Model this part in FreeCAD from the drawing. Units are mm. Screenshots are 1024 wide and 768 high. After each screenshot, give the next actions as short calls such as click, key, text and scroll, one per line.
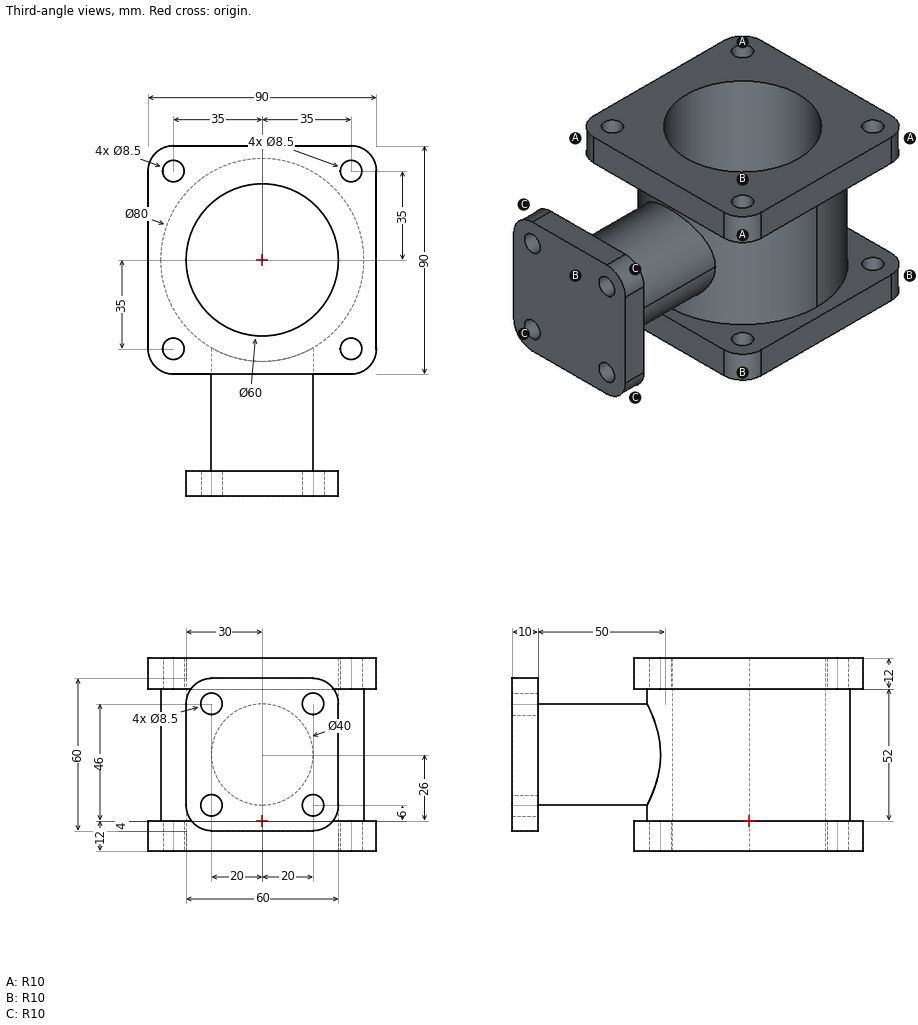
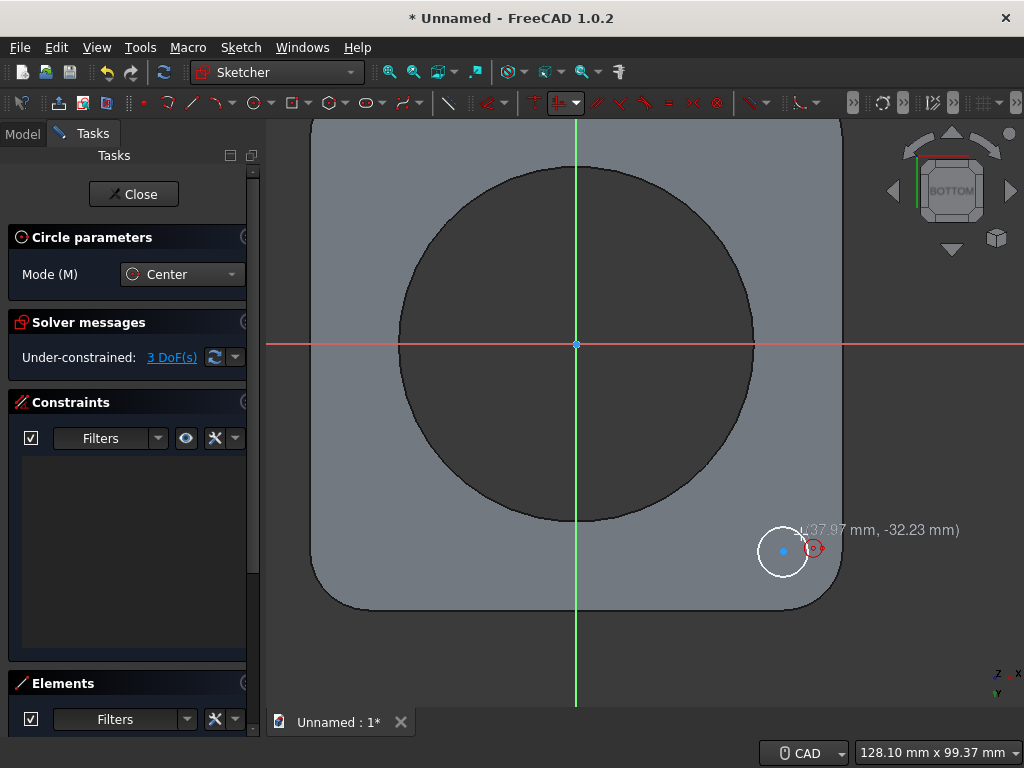
click(369, 551)
click(387, 534)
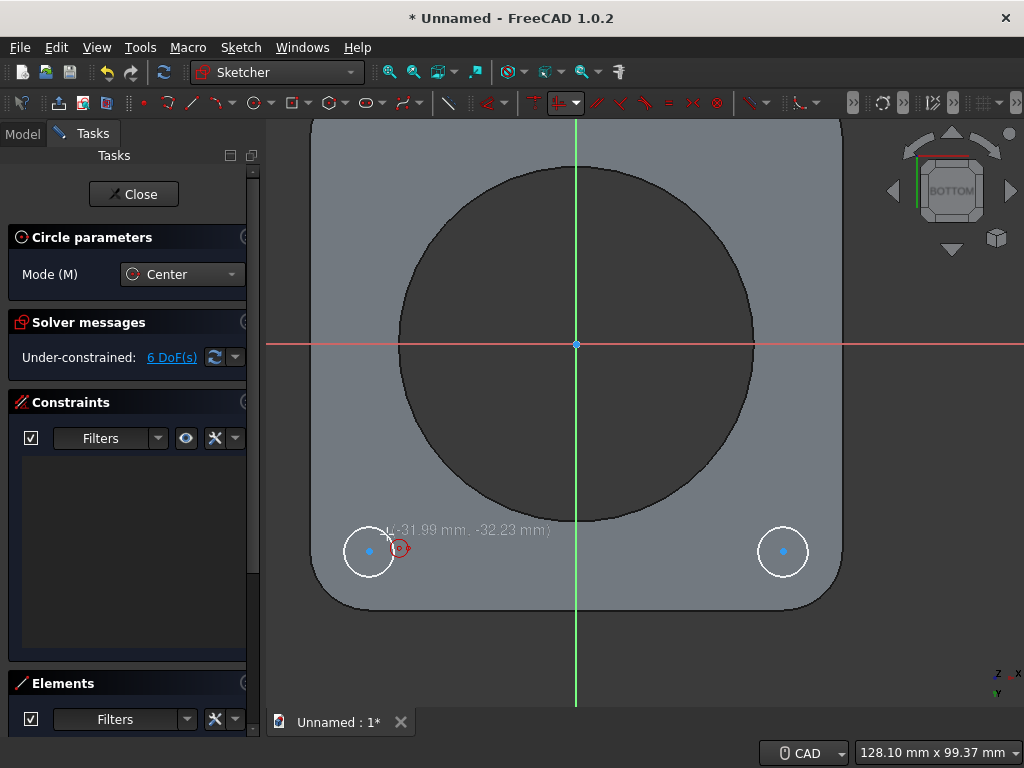
scroll(577, 679, down, 1)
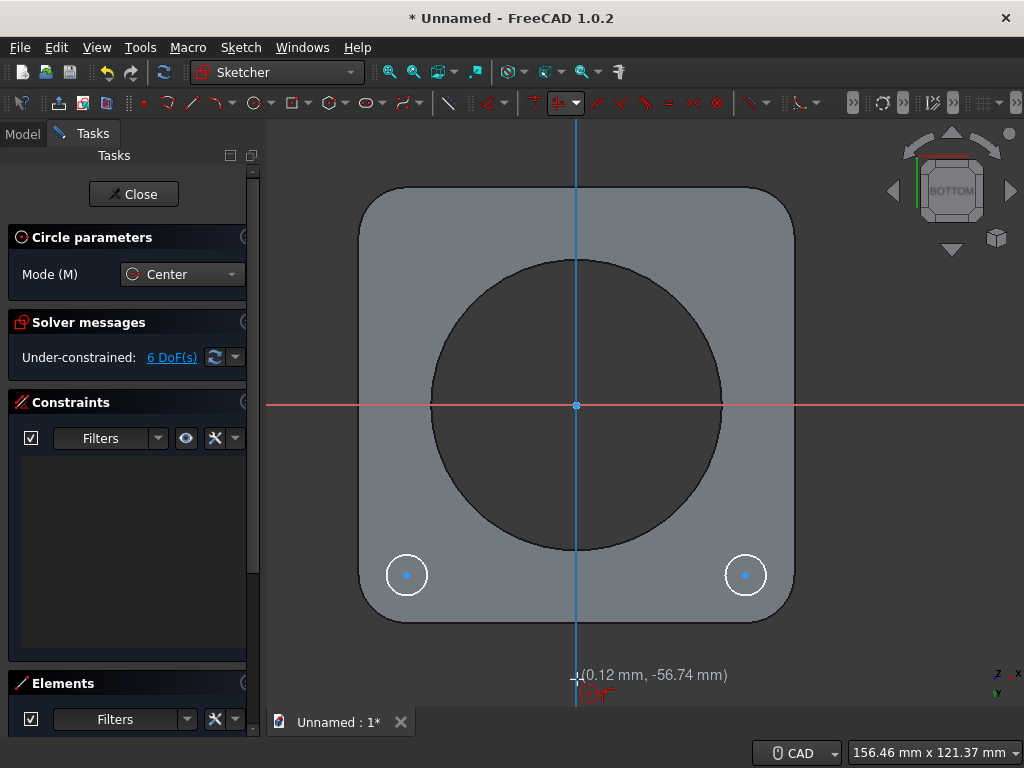
click(407, 236)
click(421, 221)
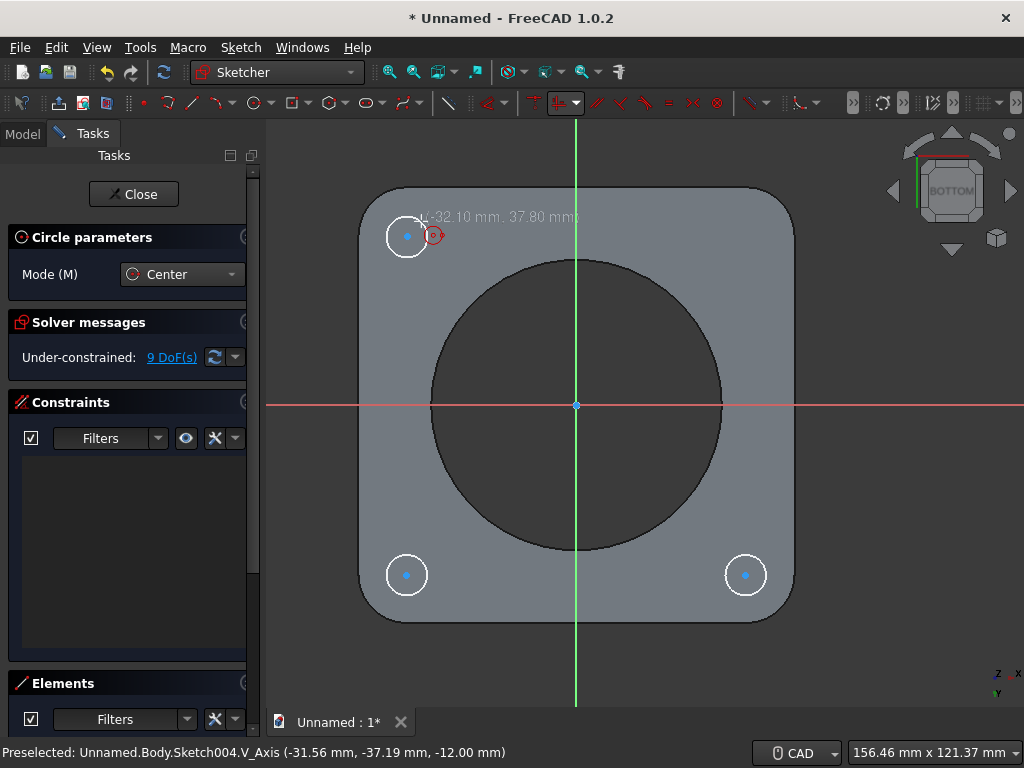
click(746, 236)
click(761, 221)
key(Escape)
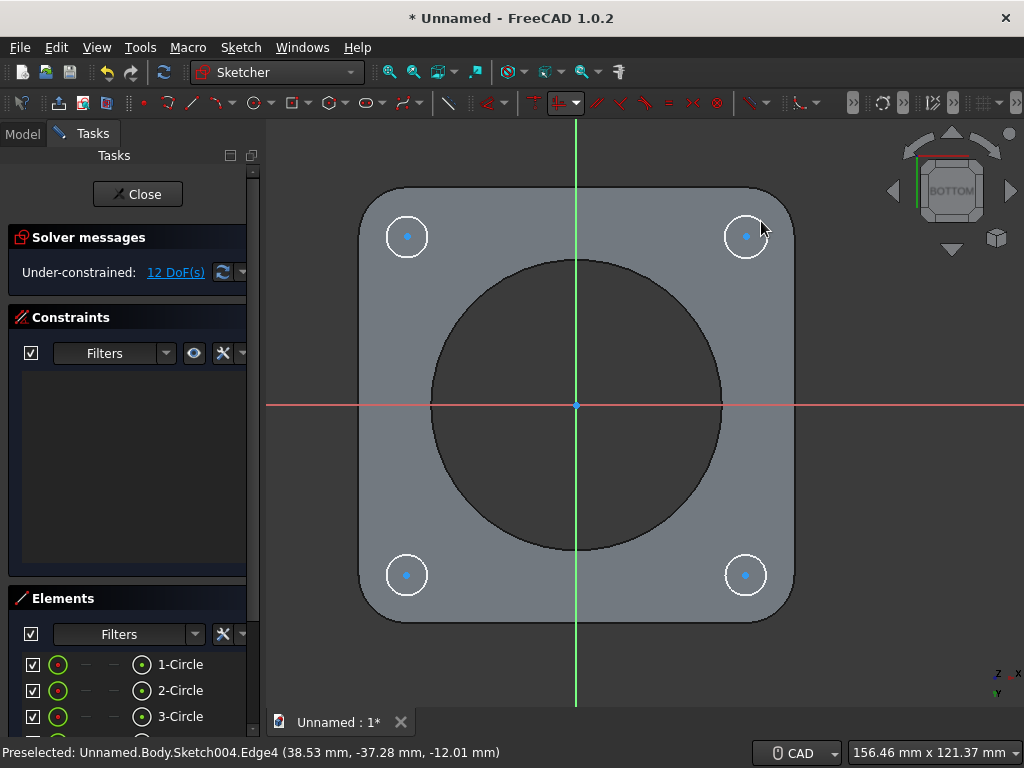
click(760, 561)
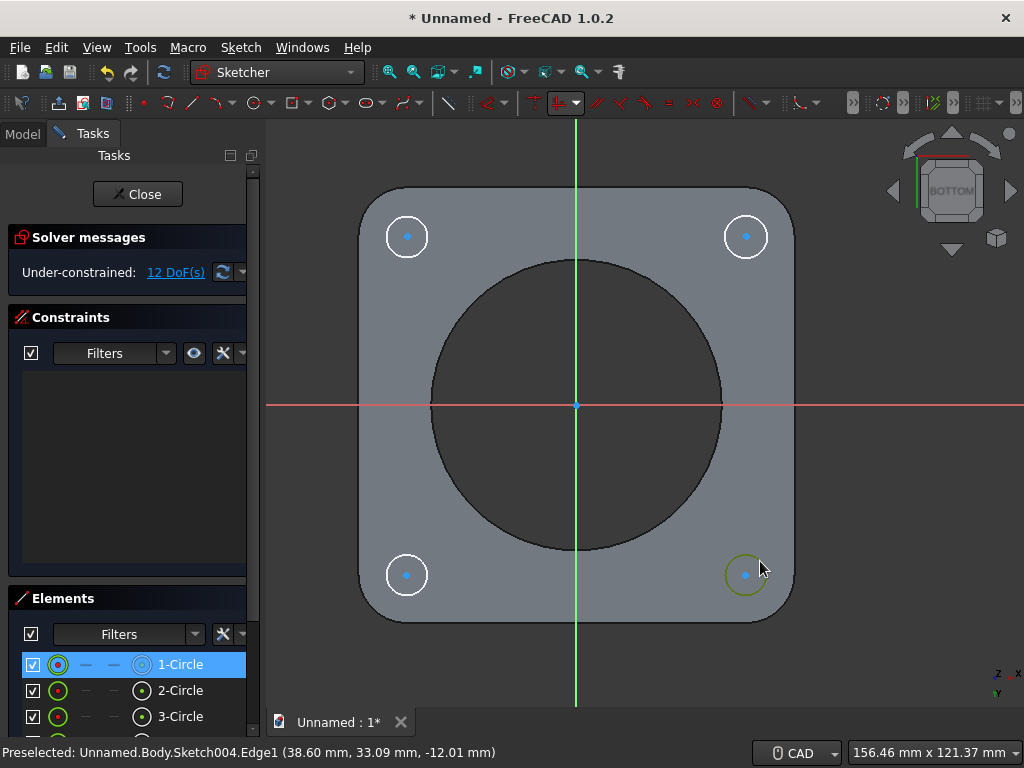
click(421, 561)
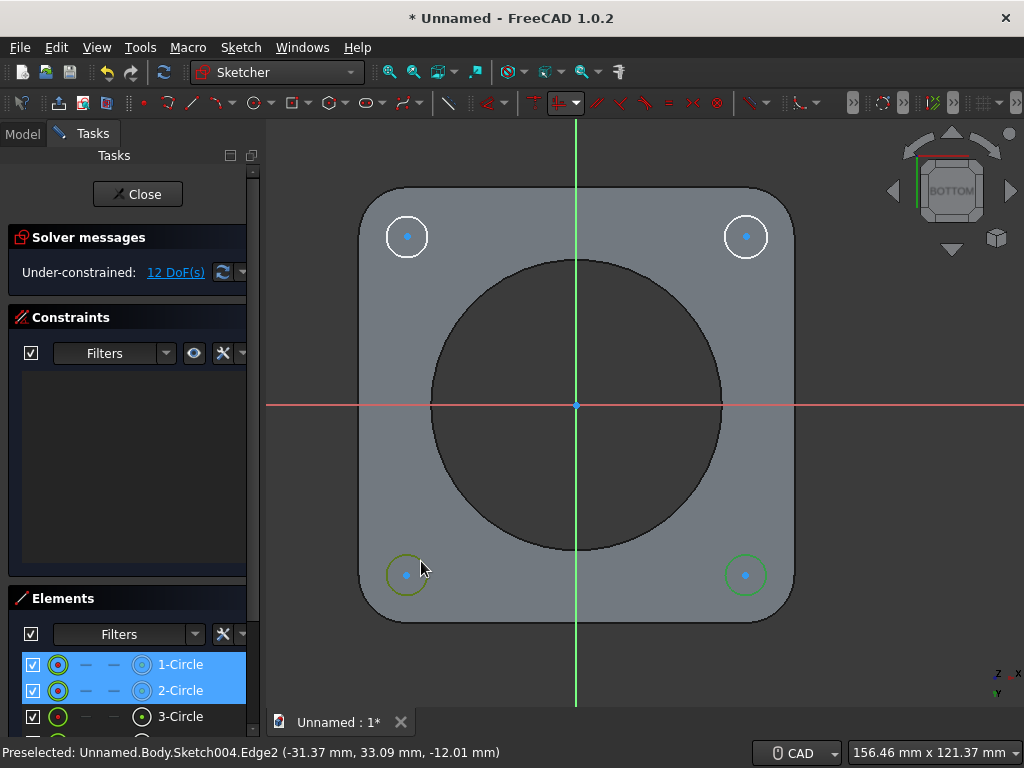
click(421, 222)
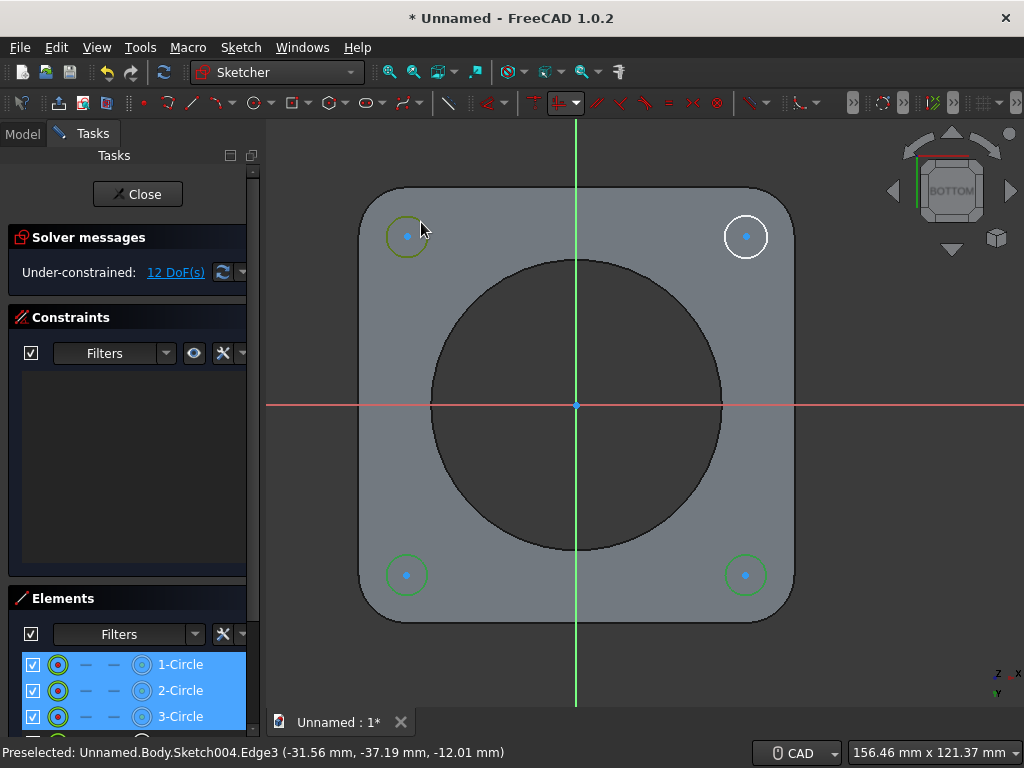
click(761, 222)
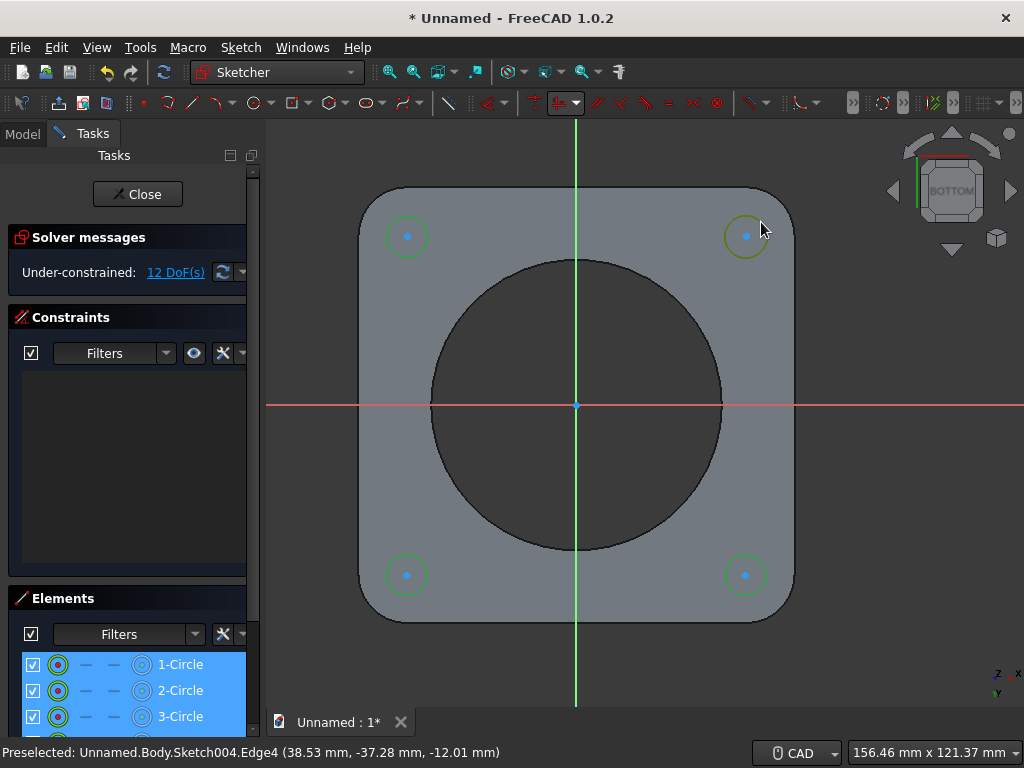
click(670, 104)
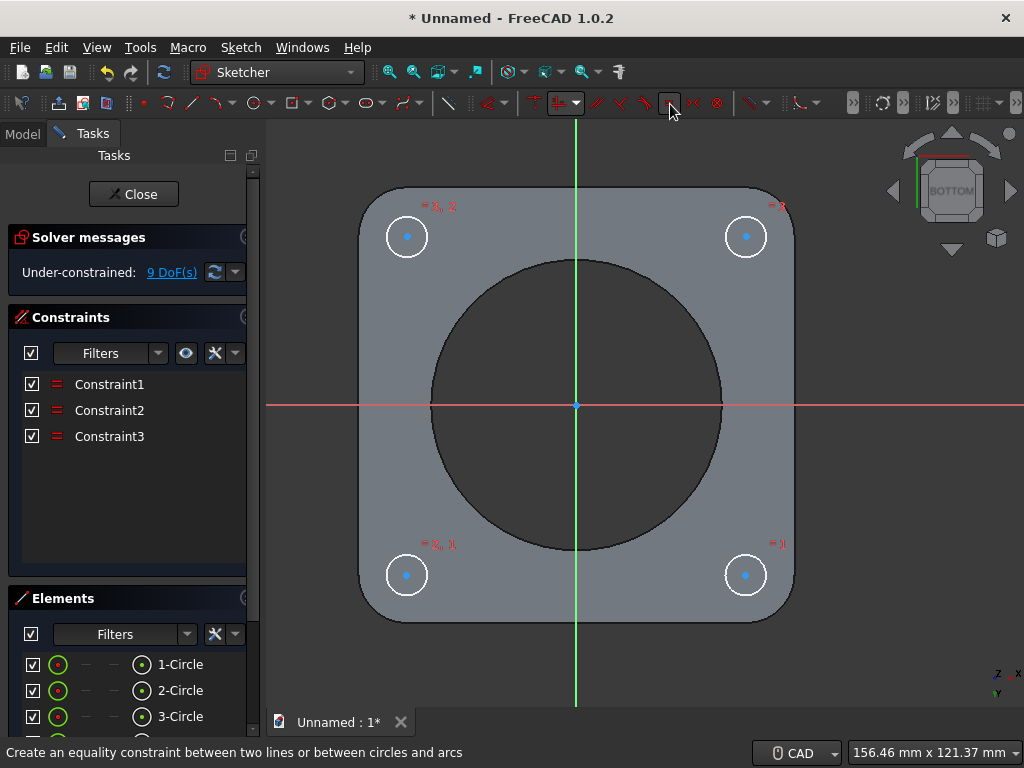
click(746, 575)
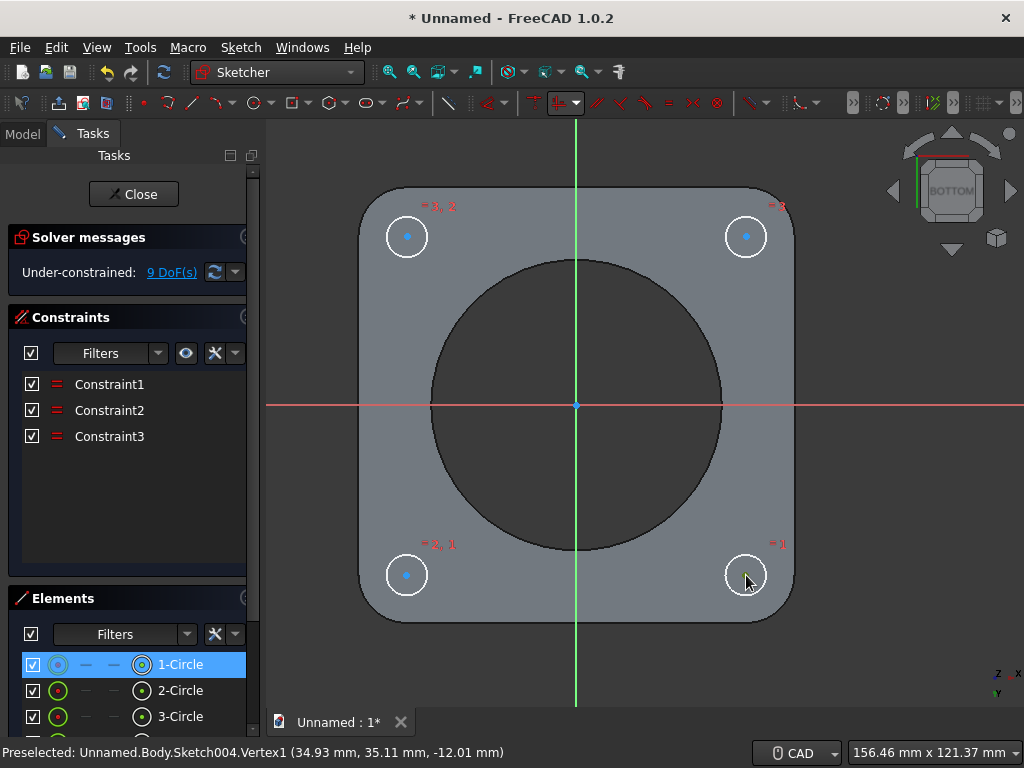
click(407, 575)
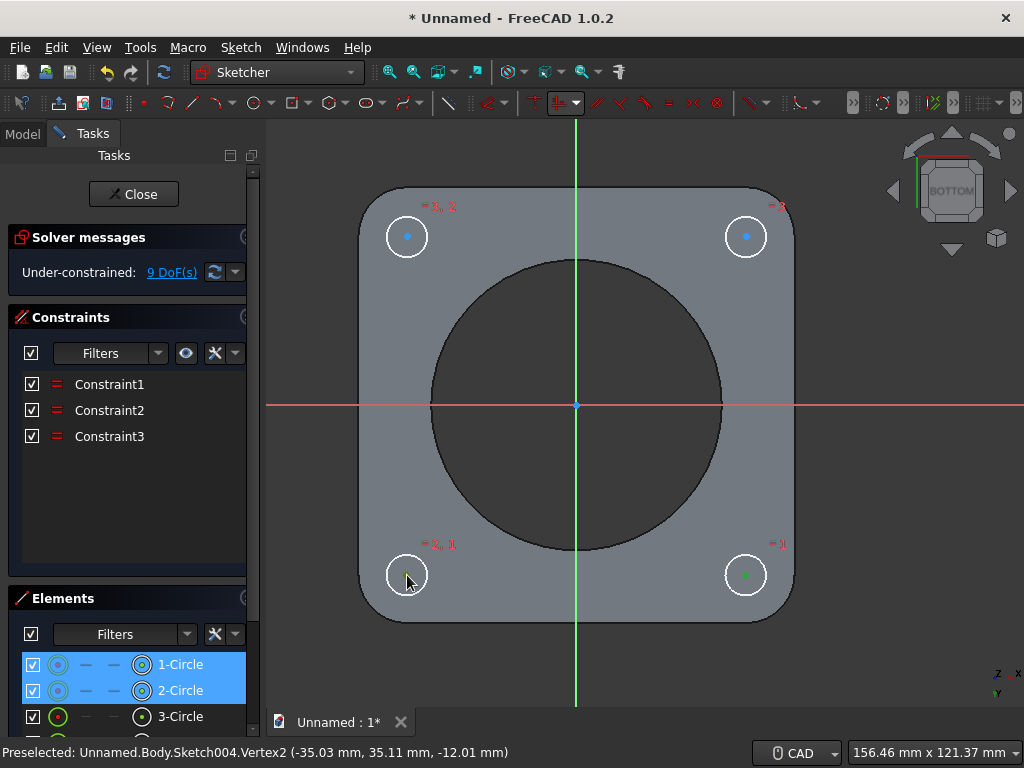
key(h)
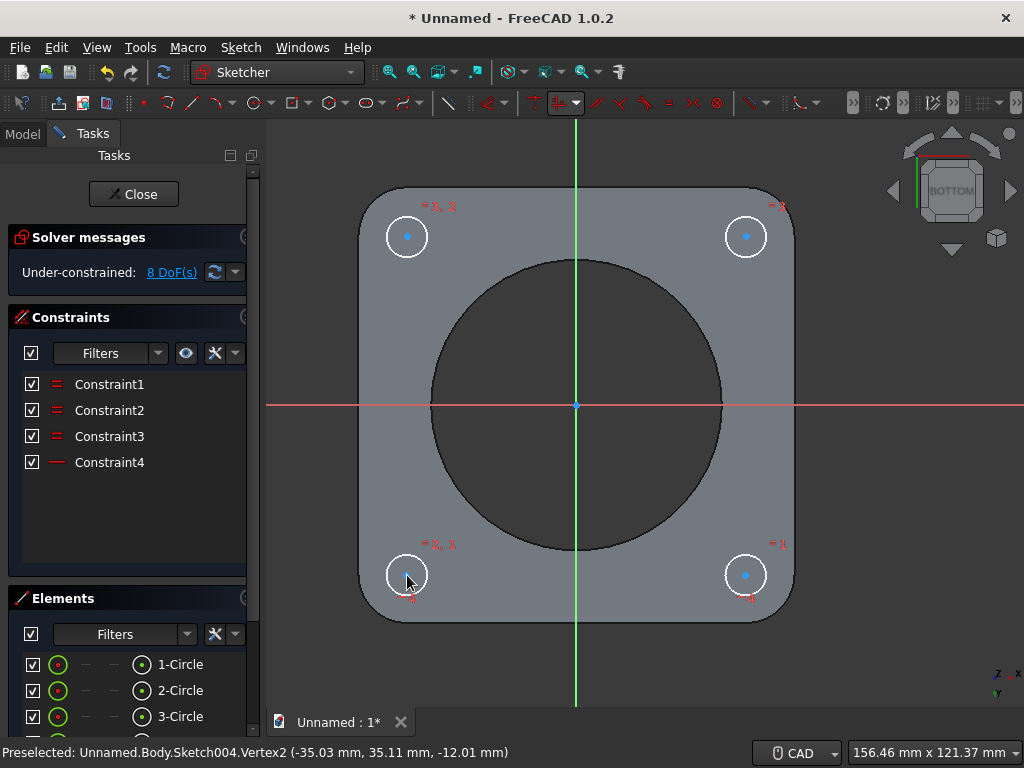
click(407, 575)